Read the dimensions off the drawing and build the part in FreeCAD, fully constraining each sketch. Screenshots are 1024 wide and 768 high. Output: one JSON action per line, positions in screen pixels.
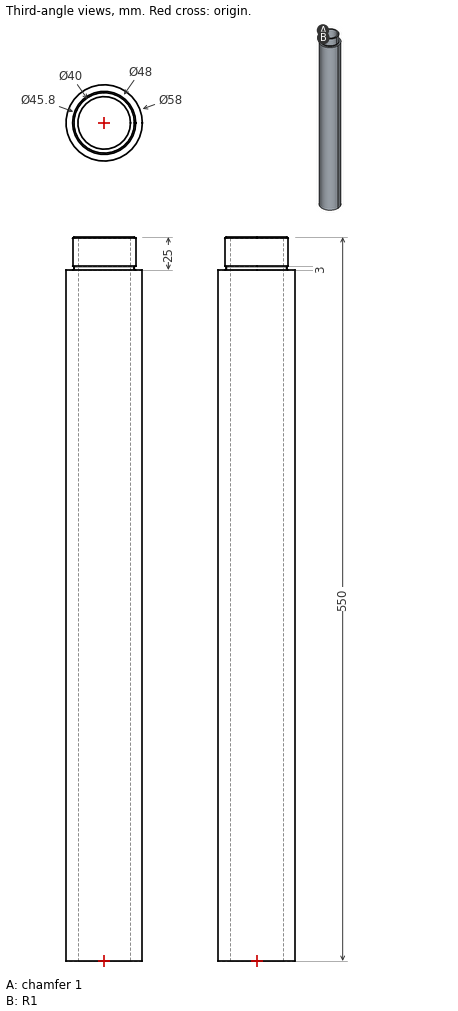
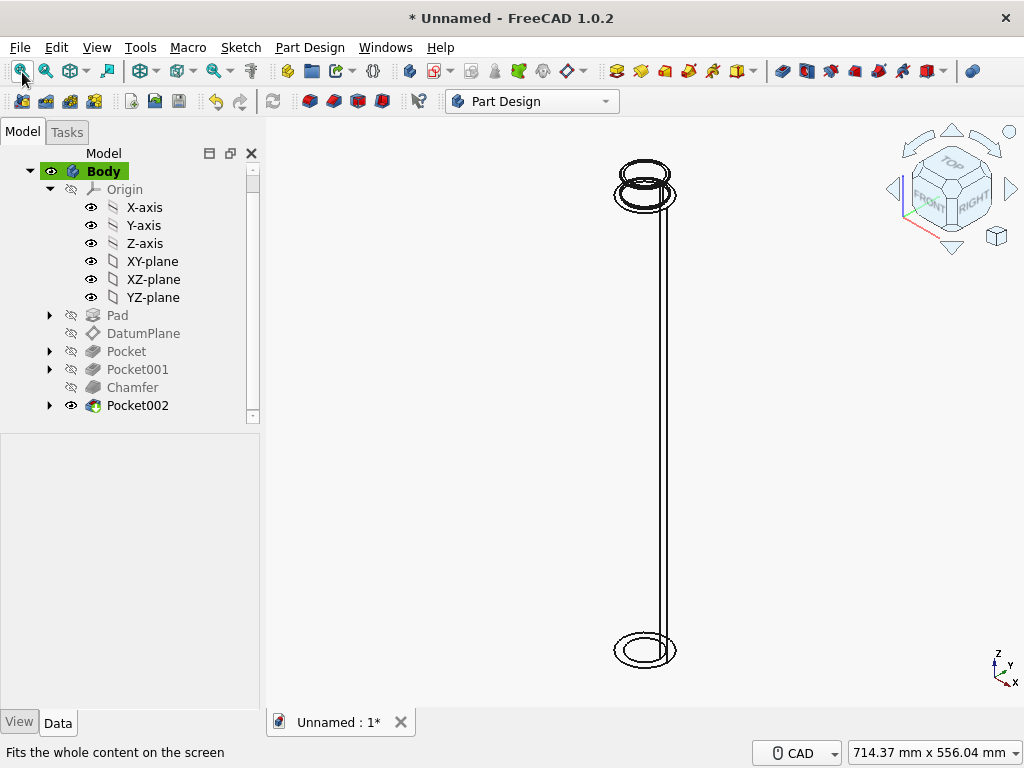
{"action": "left_click", "coordinate": [641, 178]}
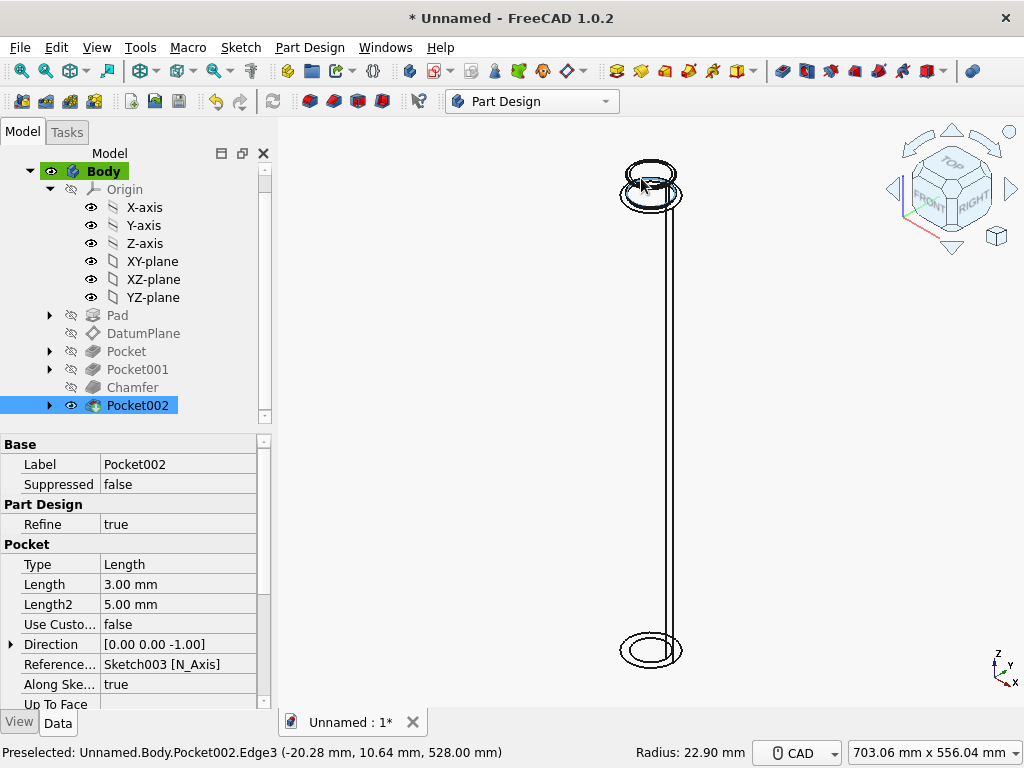
{"action": "scroll", "coordinate": [634, 184], "scroll_direction": "up", "scroll_amount": 6}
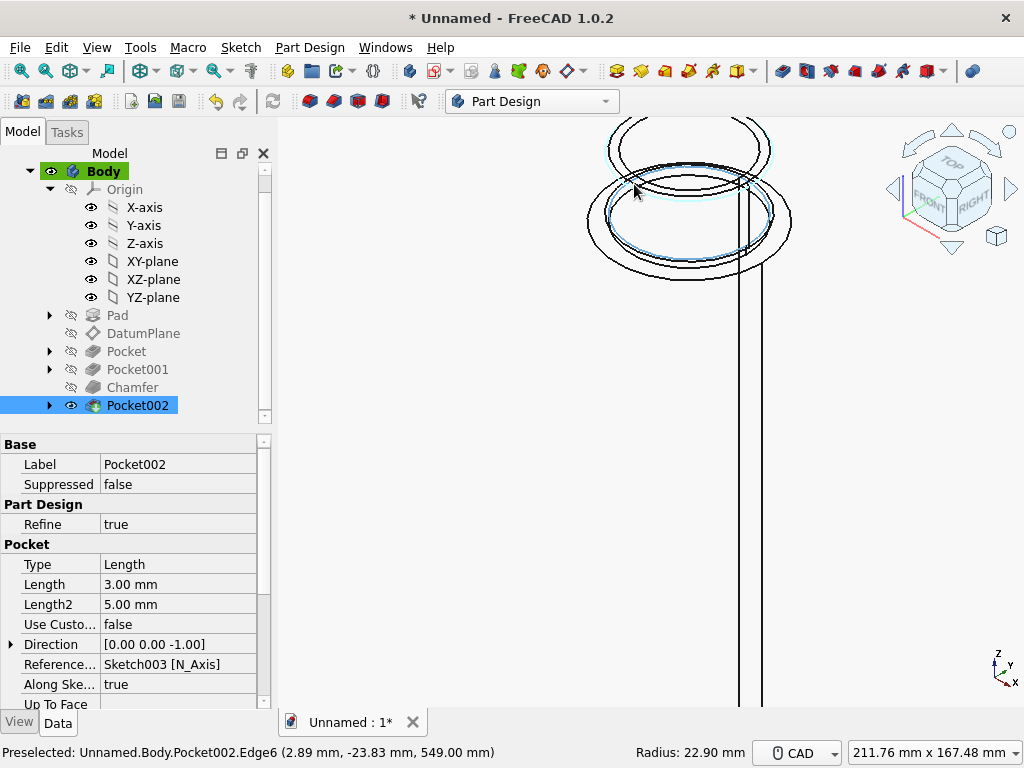
{"action": "left_click", "coordinate": [677, 175], "text": "ctrl"}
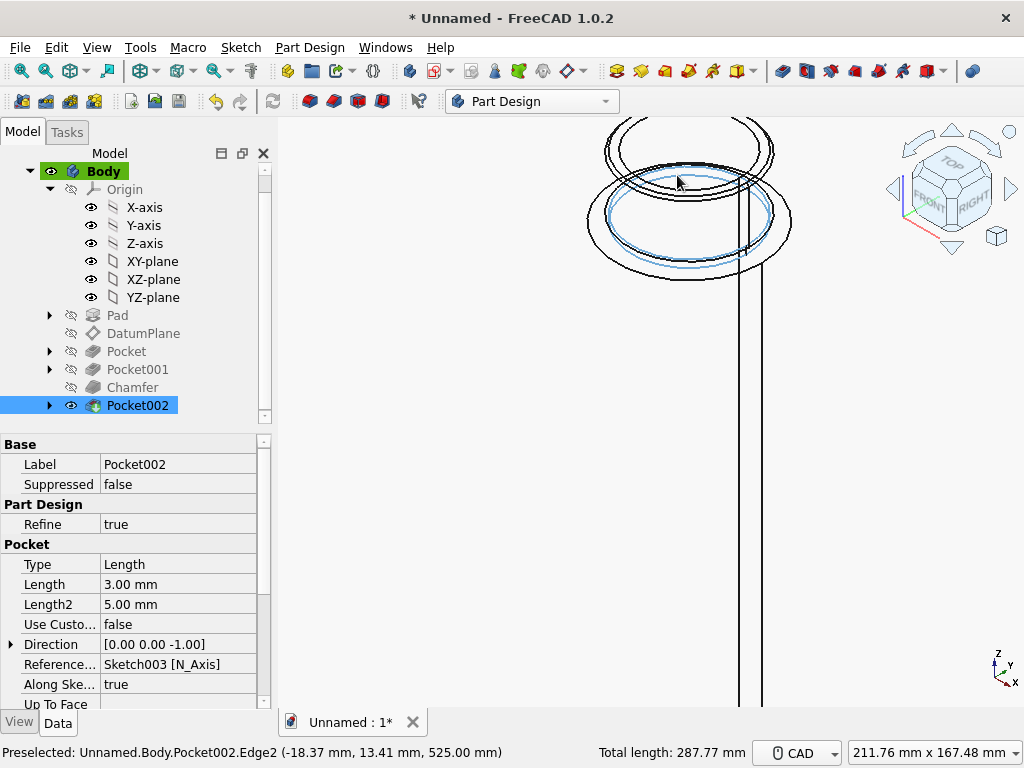
{"action": "key", "text": "v 1"}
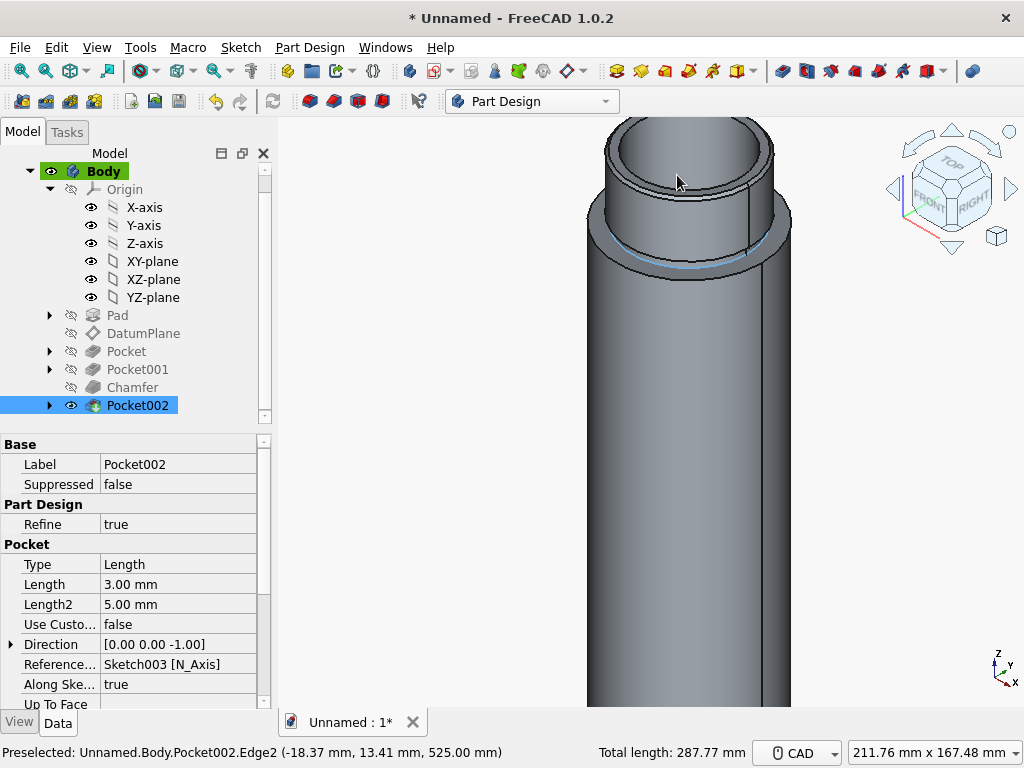
{"action": "left_click", "coordinate": [310, 102]}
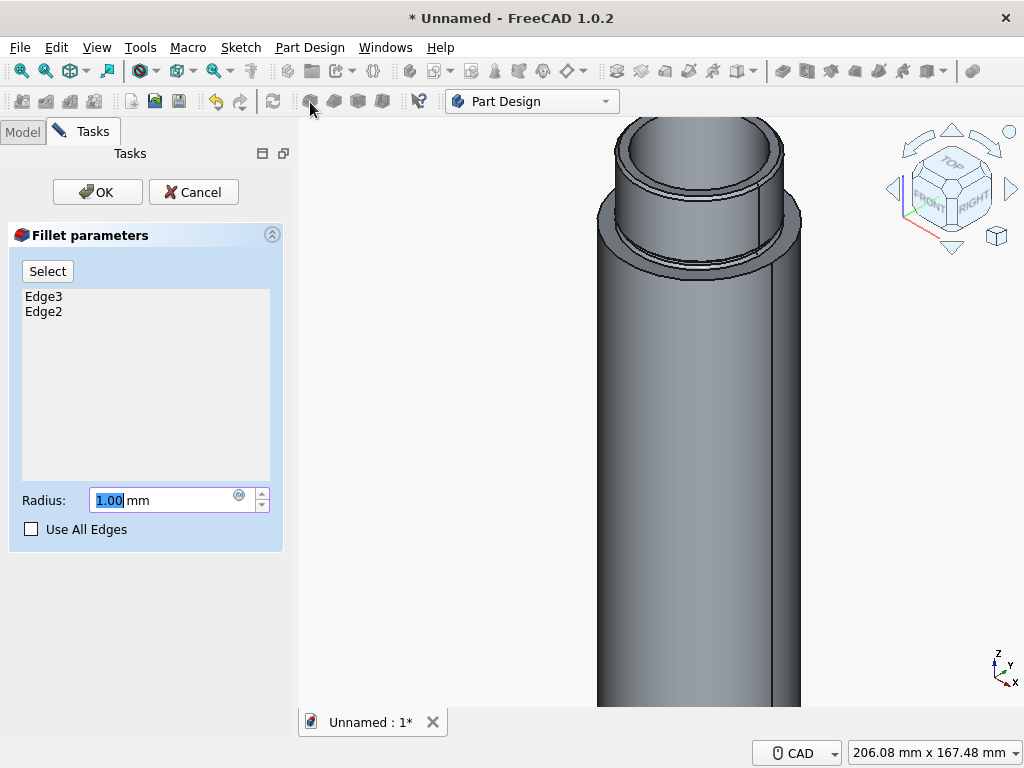
{"action": "type", "text": "1"}
{"action": "key", "text": "Tab"}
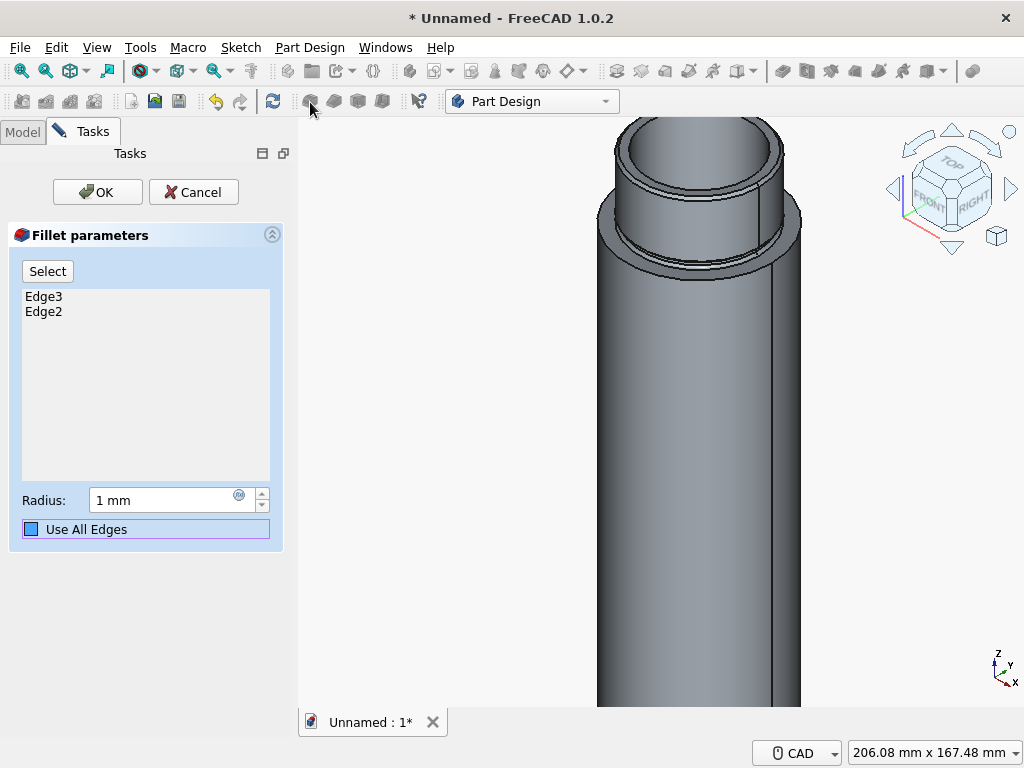
{"action": "left_click", "coordinate": [98, 192]}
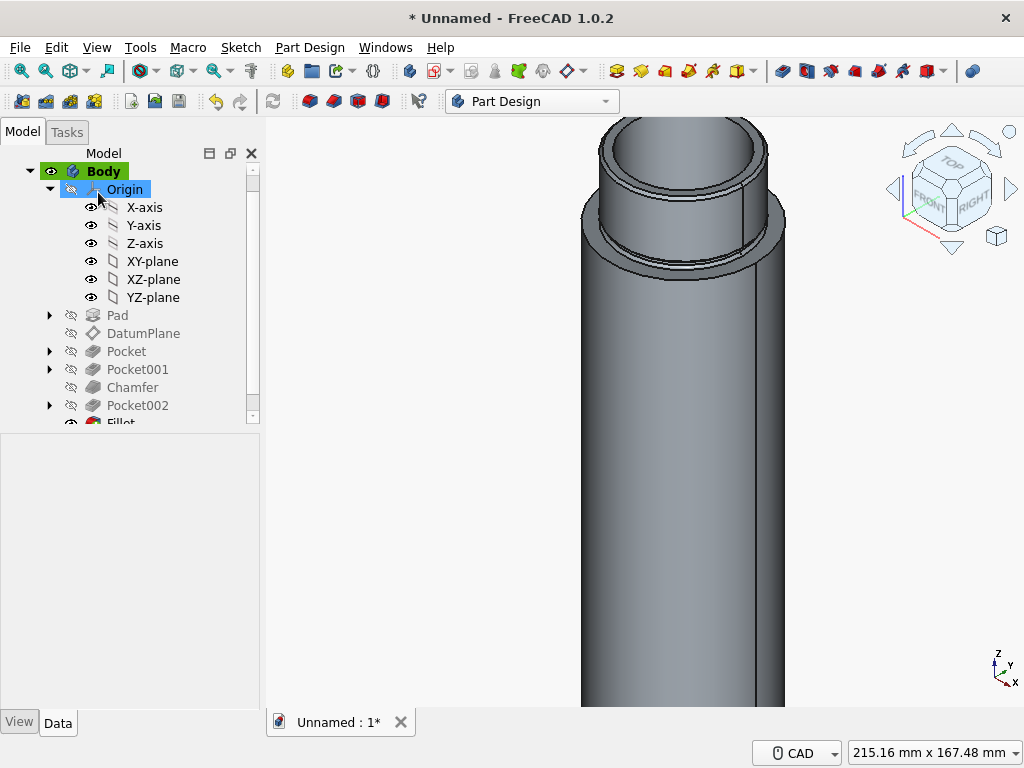
{"action": "left_click", "coordinate": [22, 72]}